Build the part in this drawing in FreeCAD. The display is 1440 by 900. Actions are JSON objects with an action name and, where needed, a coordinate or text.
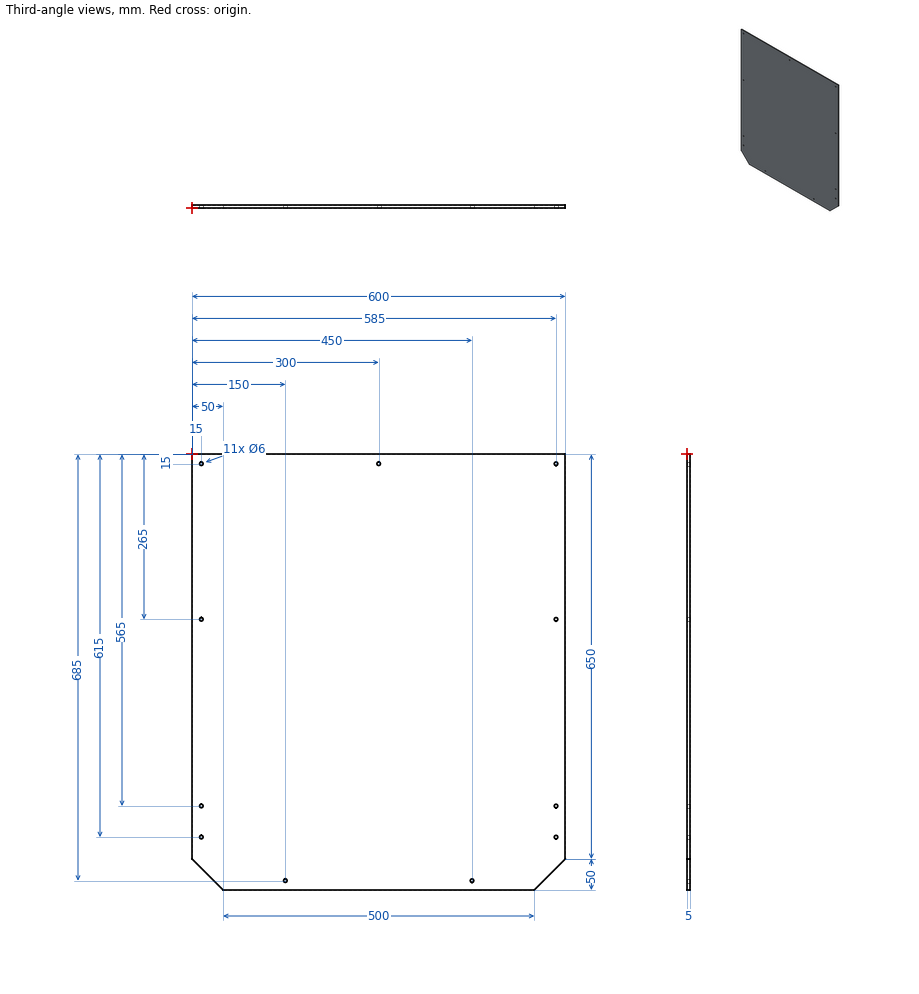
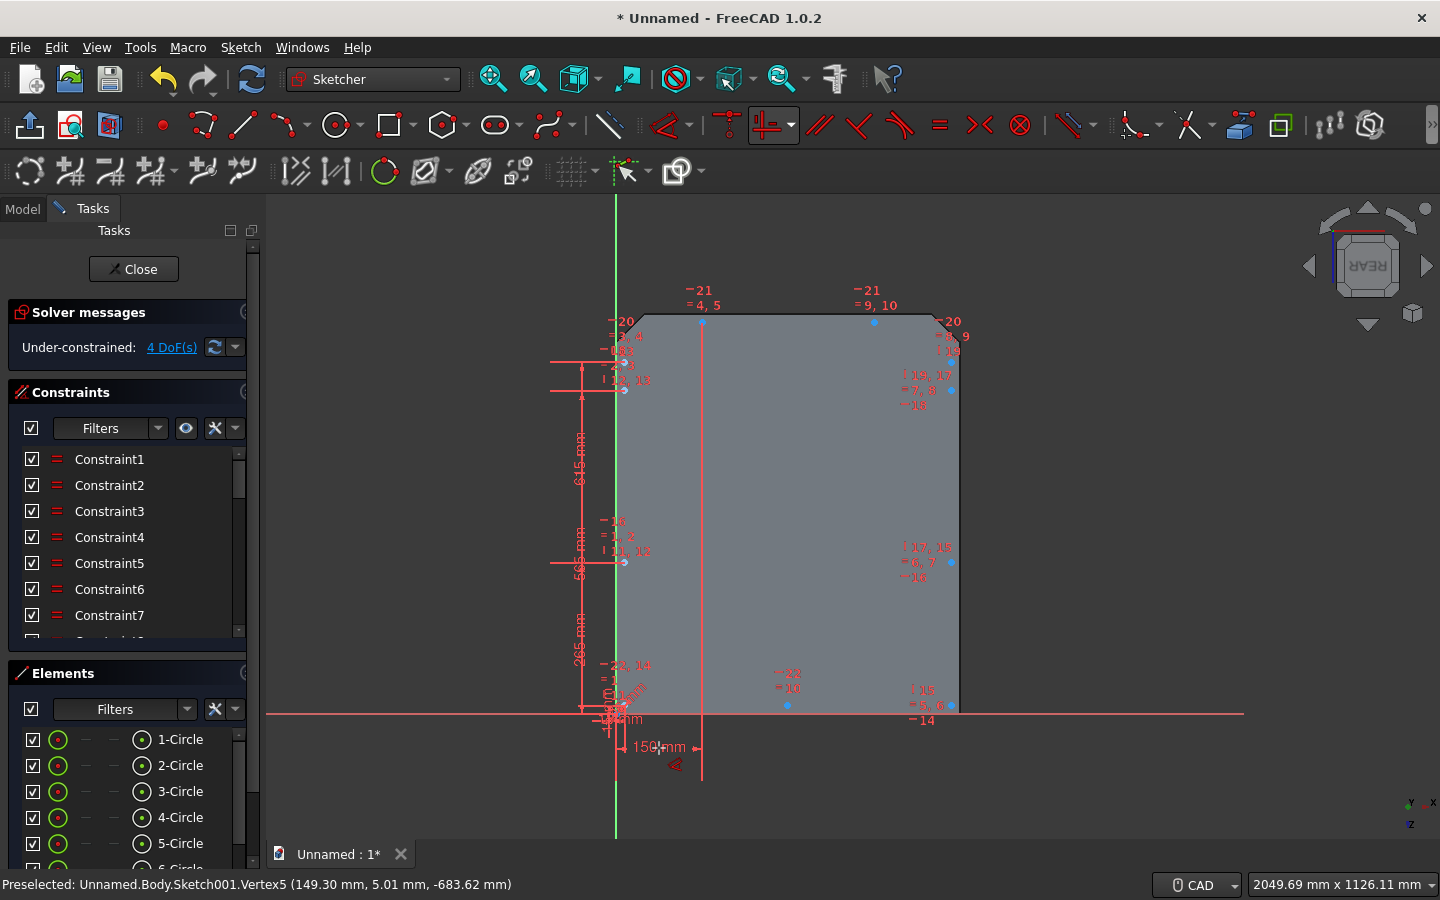
{"action": "left_click", "coordinate": [702, 323]}
{"action": "left_click", "coordinate": [582, 519]}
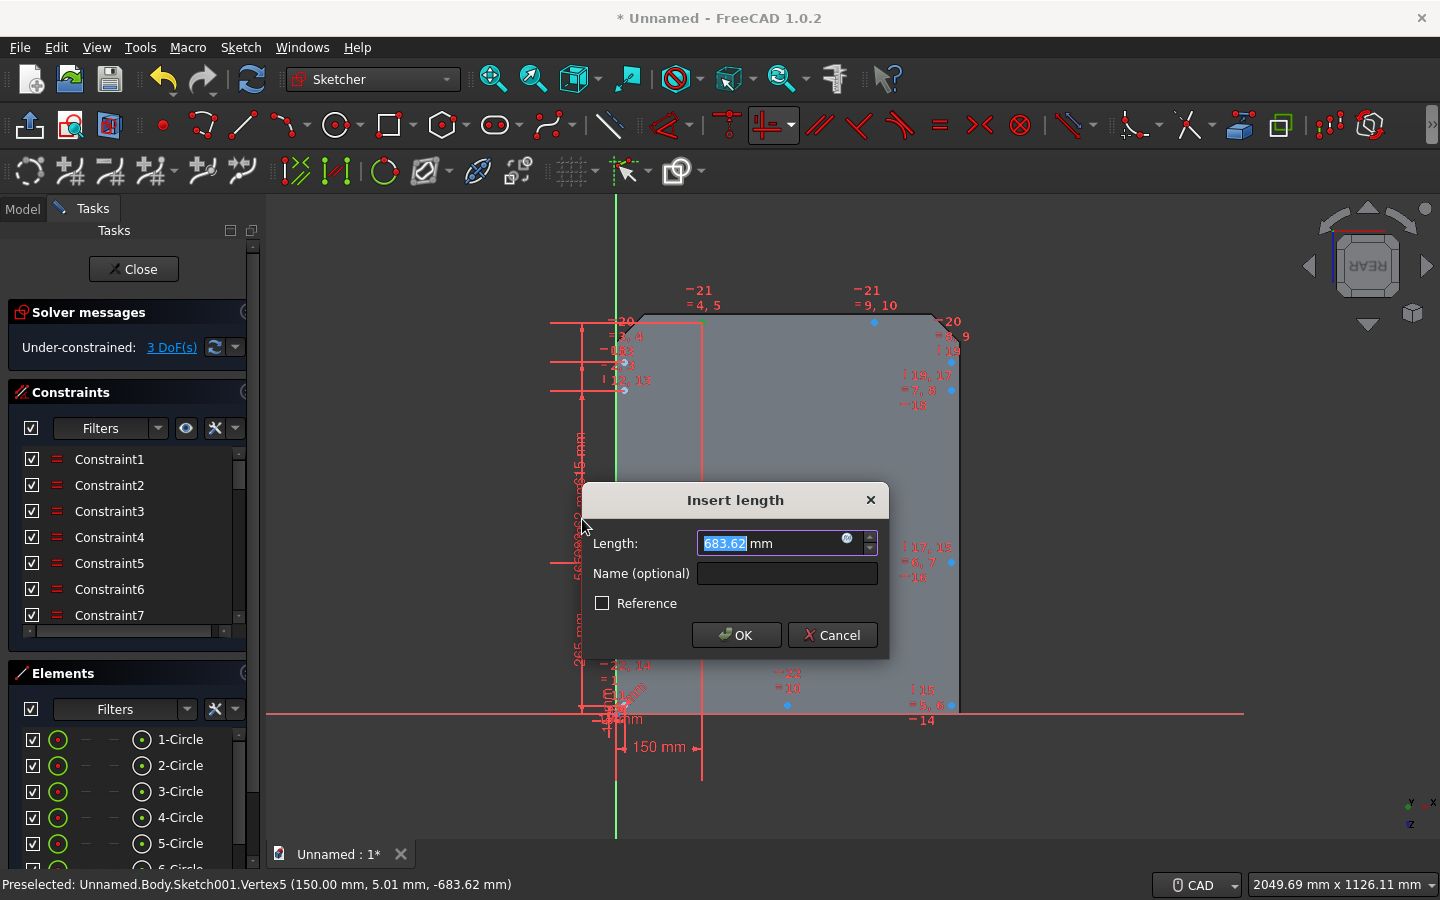
{"action": "type", "text": "685"}
{"action": "key", "text": "Return"}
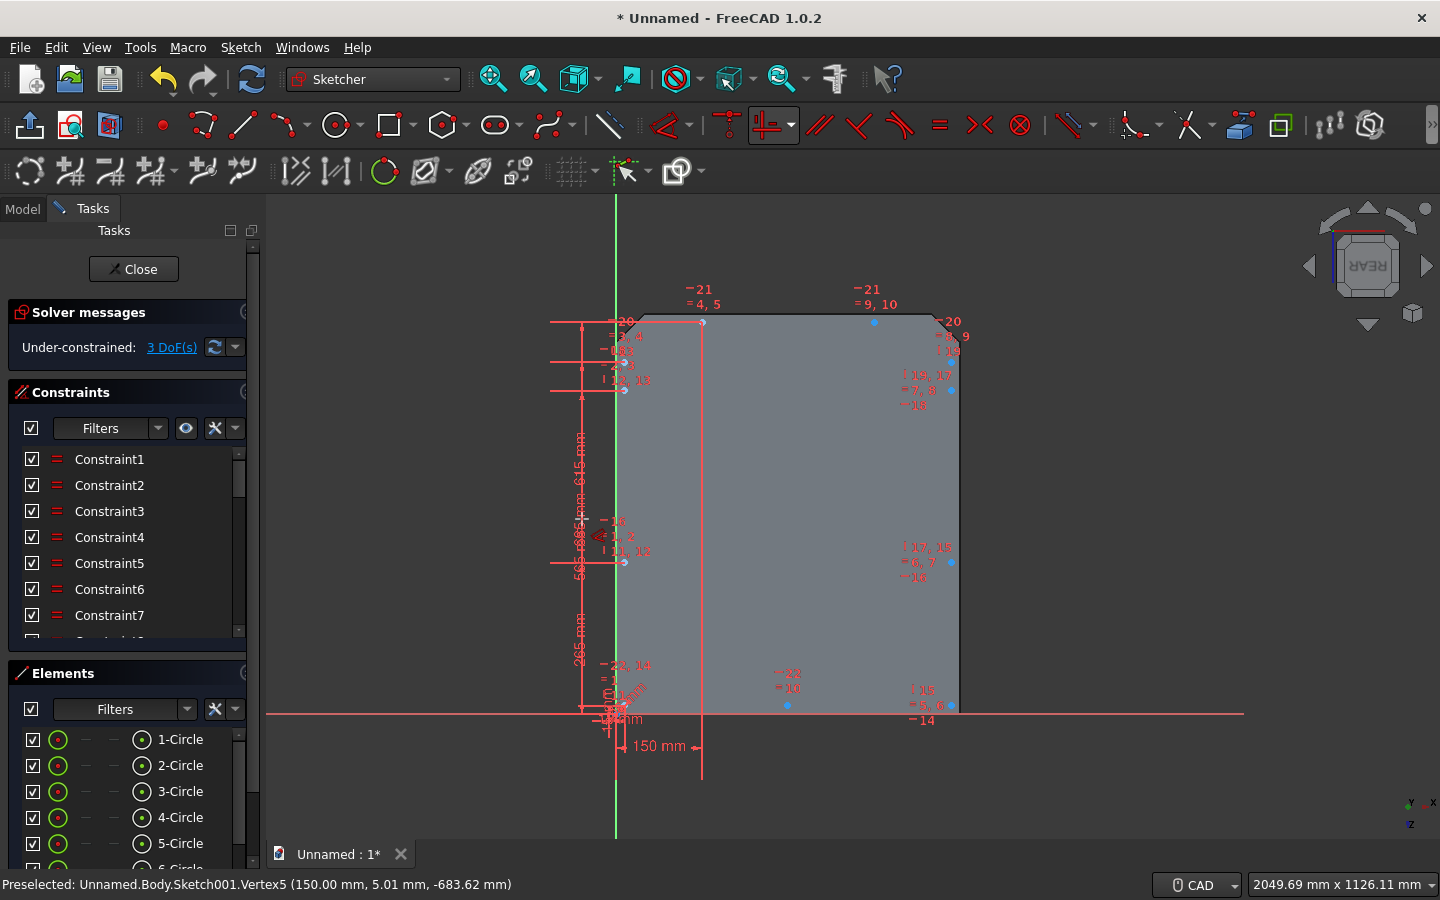
{"action": "left_click", "coordinate": [951, 706]}
{"action": "left_click", "coordinate": [784, 748]}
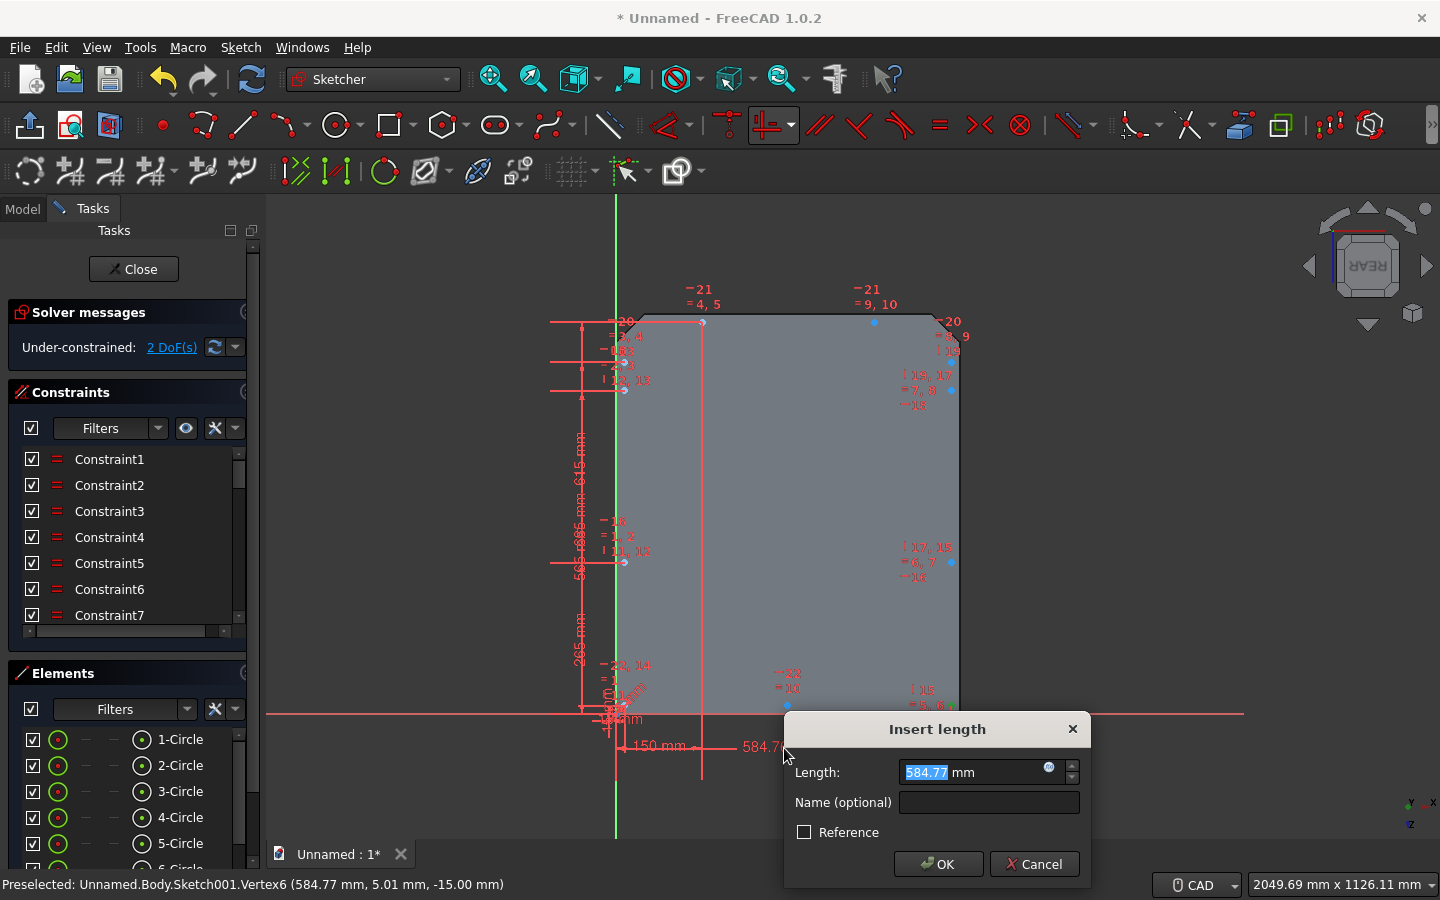
{"action": "type", "text": "585"}
{"action": "key", "text": "Return"}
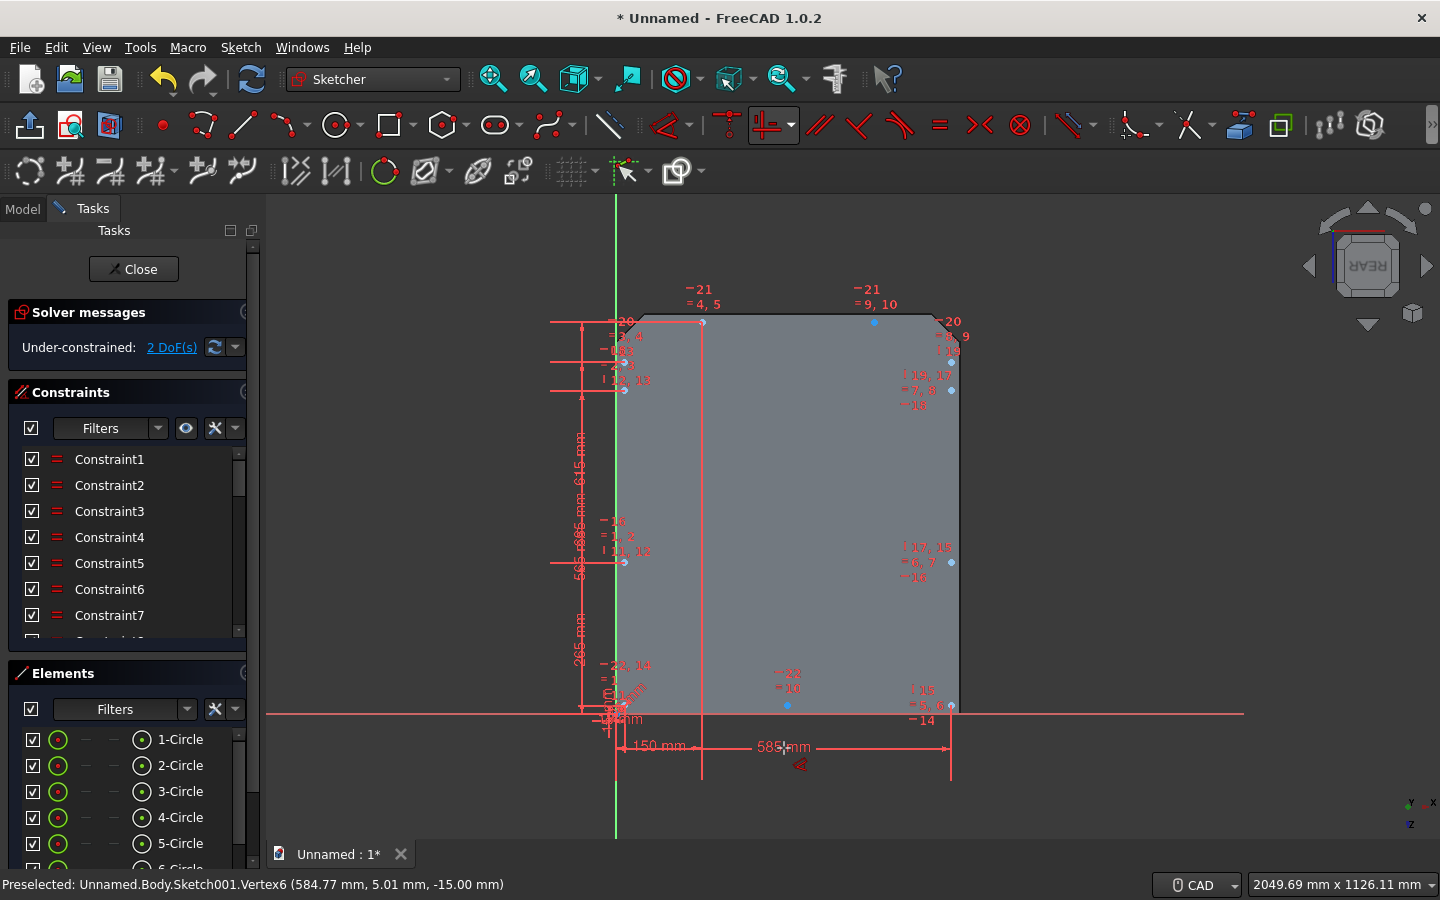
{"action": "left_click", "coordinate": [874, 322]}
{"action": "left_click", "coordinate": [745, 288]}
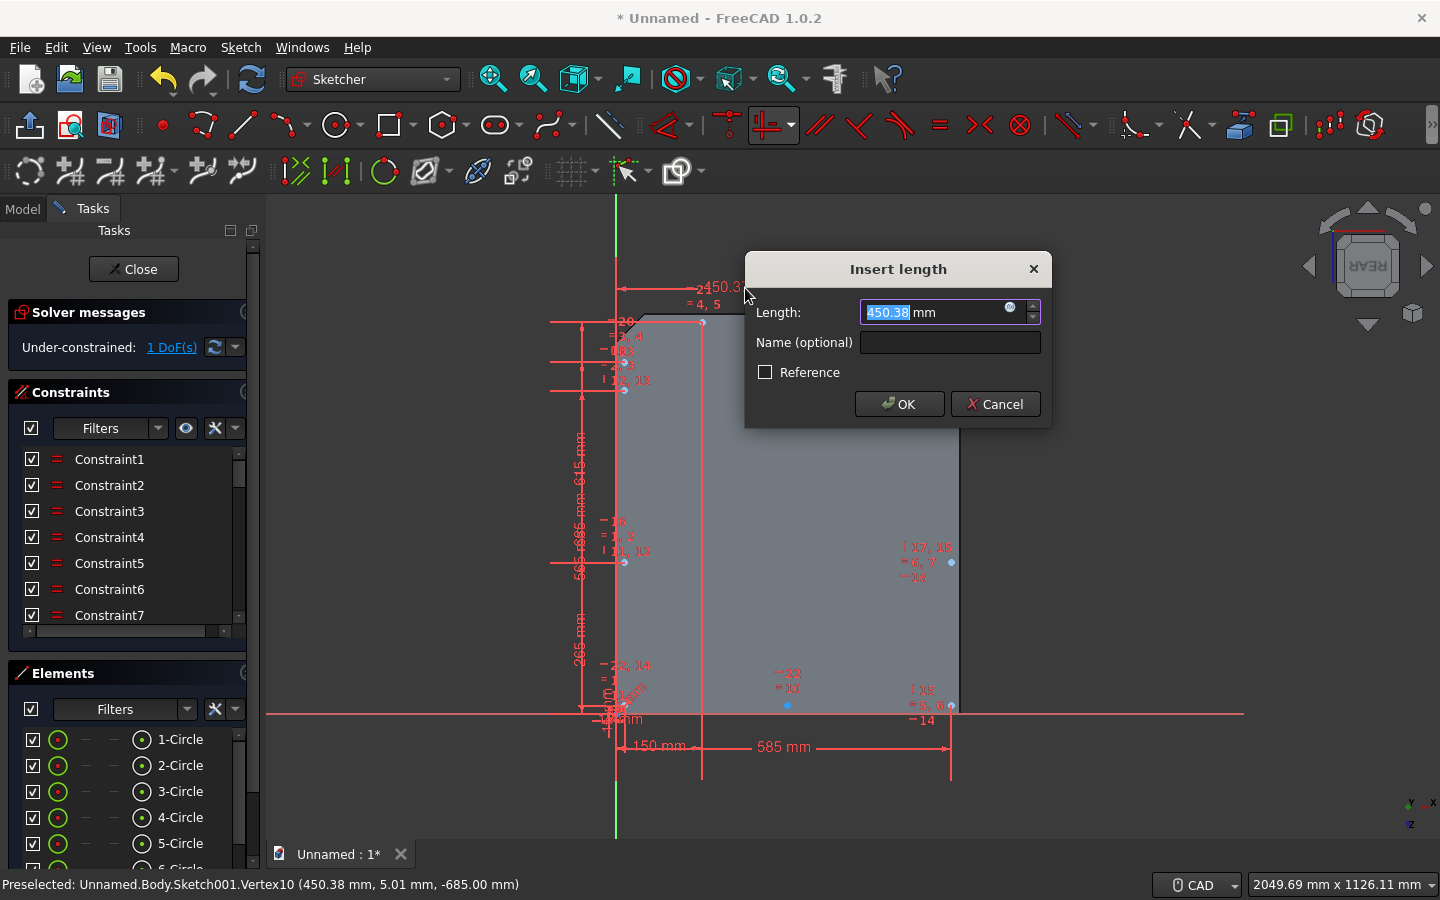
{"action": "type", "text": "450"}
{"action": "key", "text": "Return"}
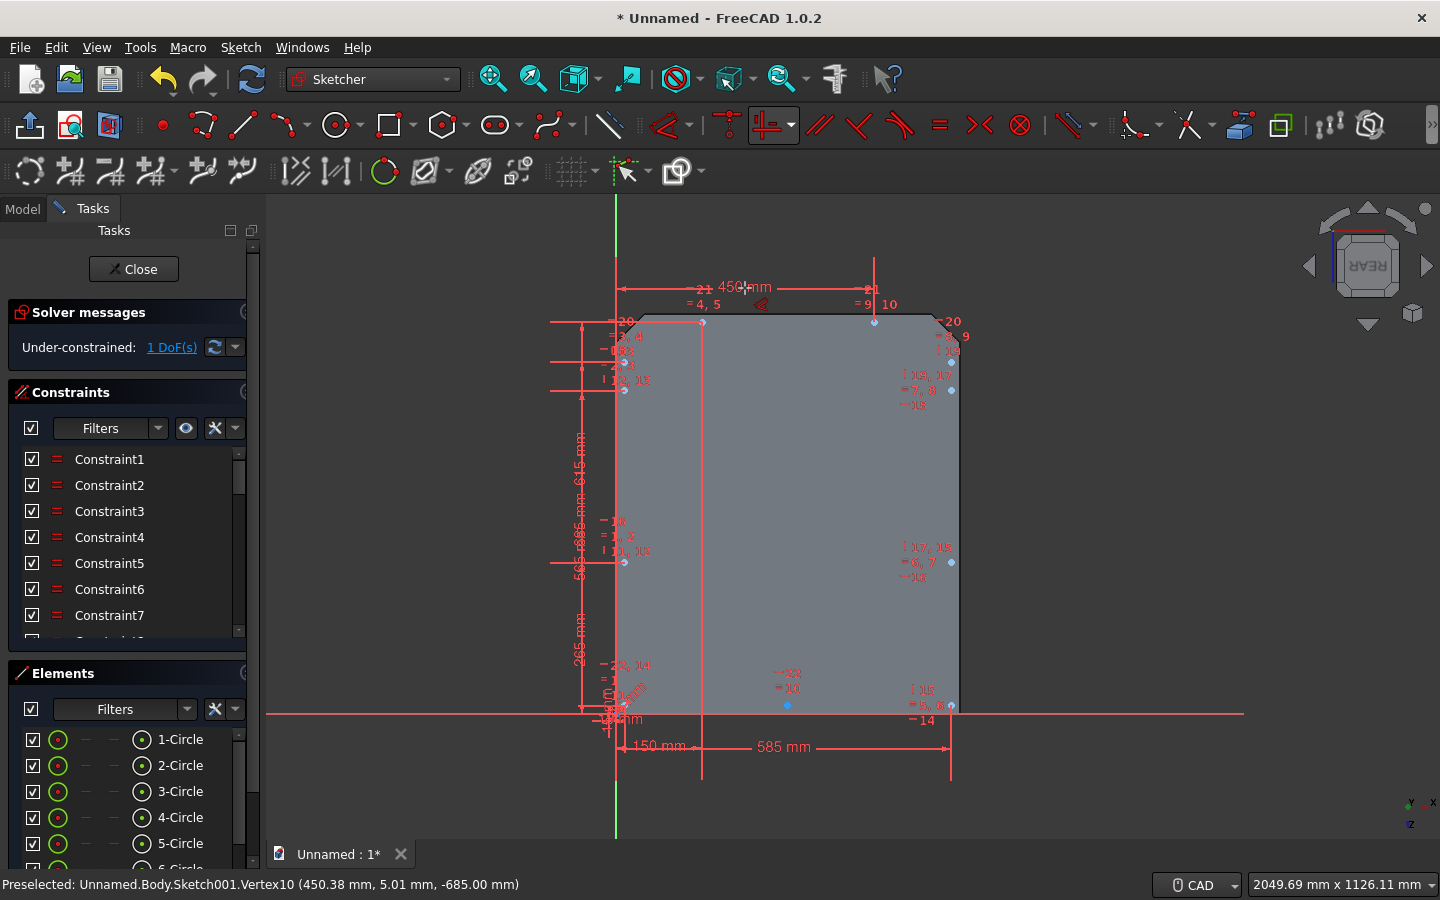
{"action": "left_click", "coordinate": [788, 706]}
{"action": "left_click", "coordinate": [702, 672]}